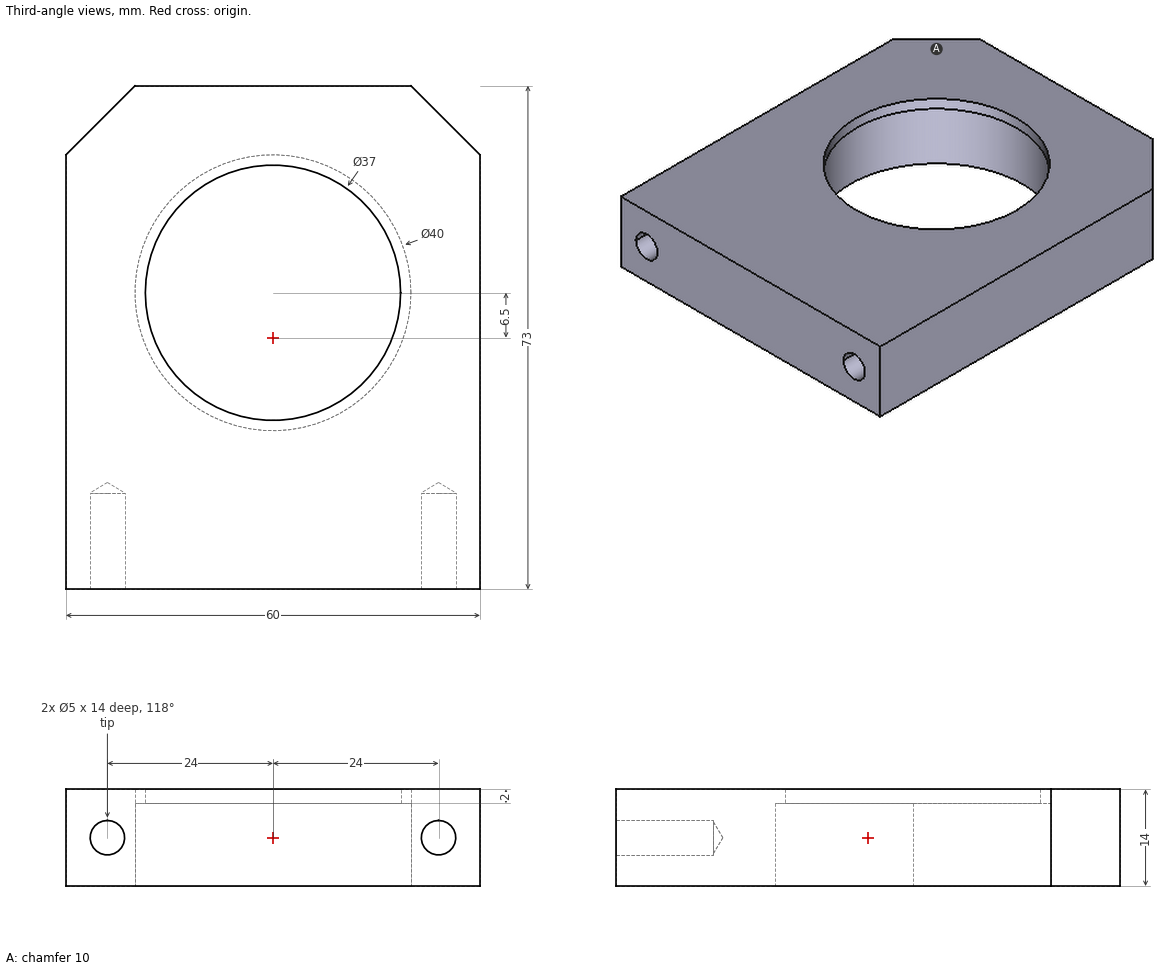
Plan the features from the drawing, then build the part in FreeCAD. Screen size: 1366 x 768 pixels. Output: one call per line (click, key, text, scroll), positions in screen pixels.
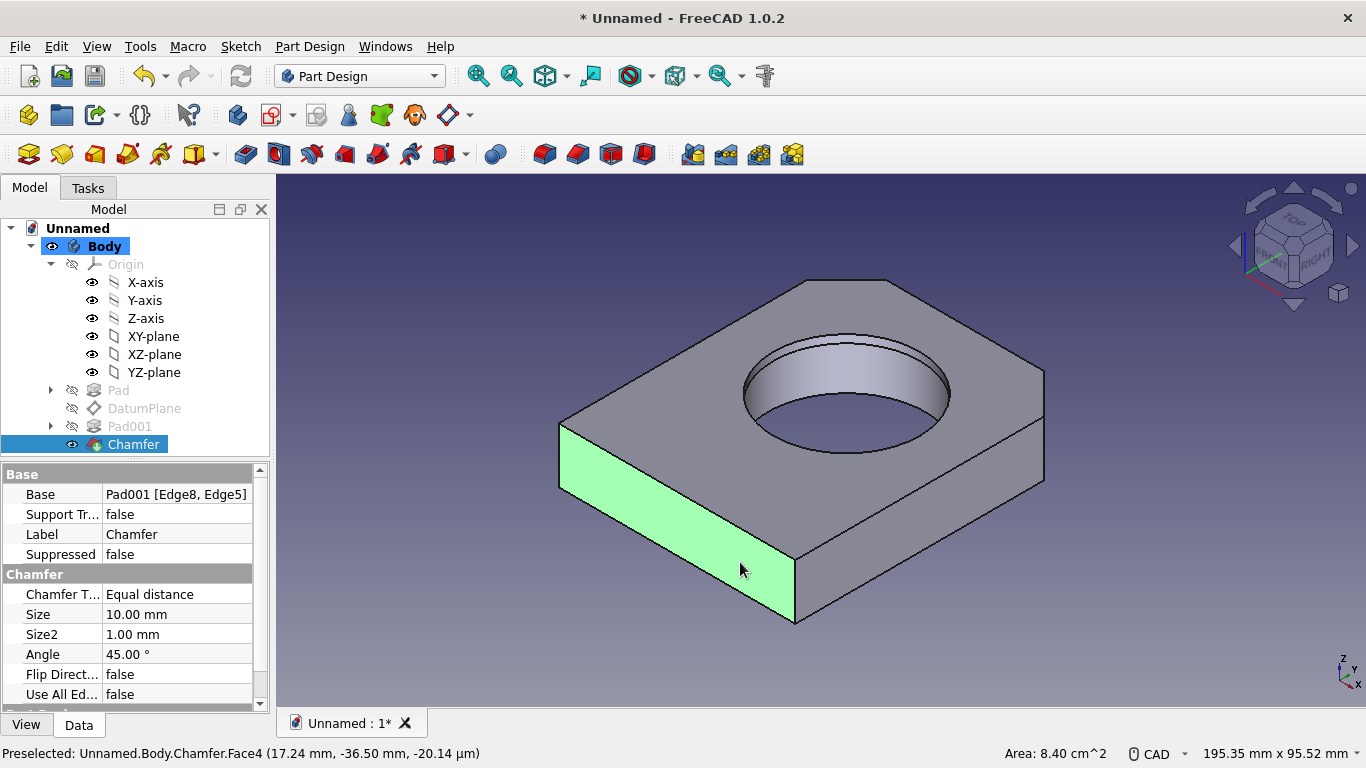
click(270, 116)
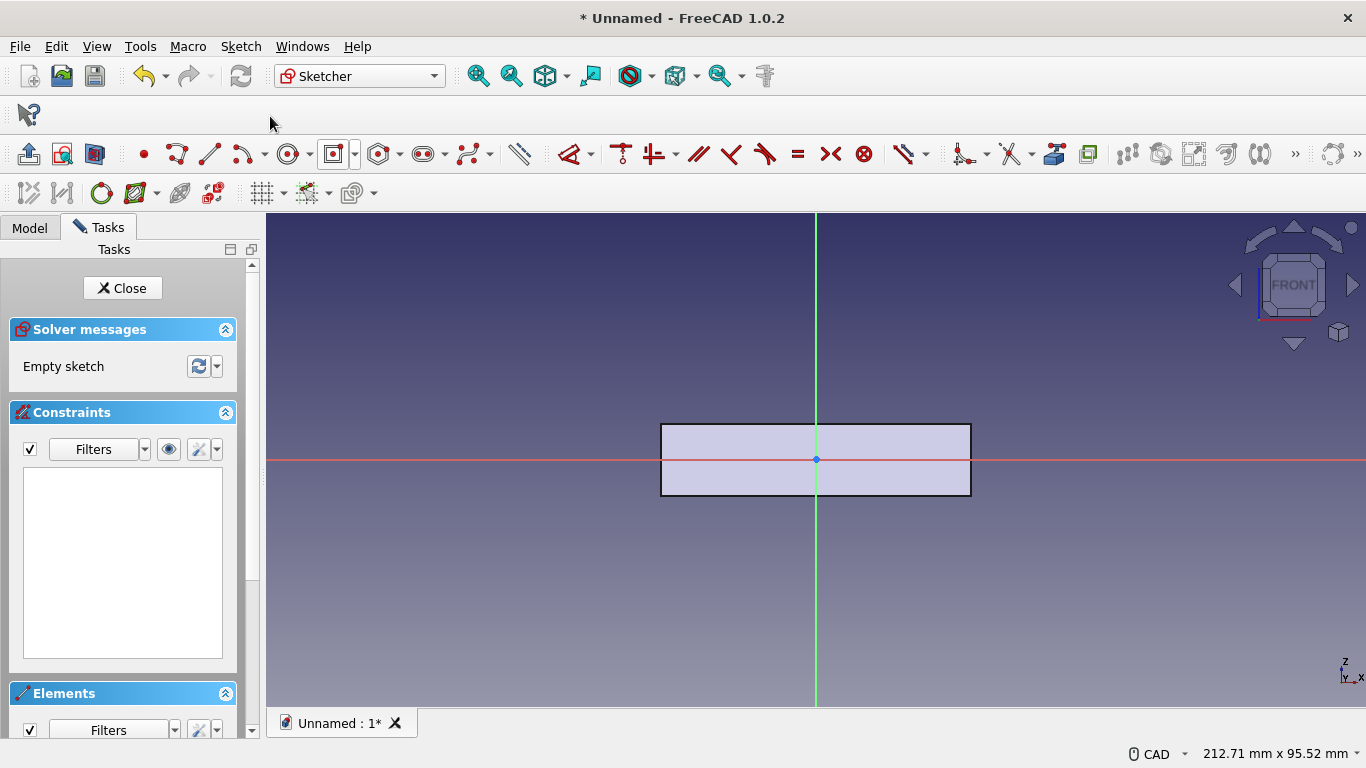
scroll(872, 460, up, 4)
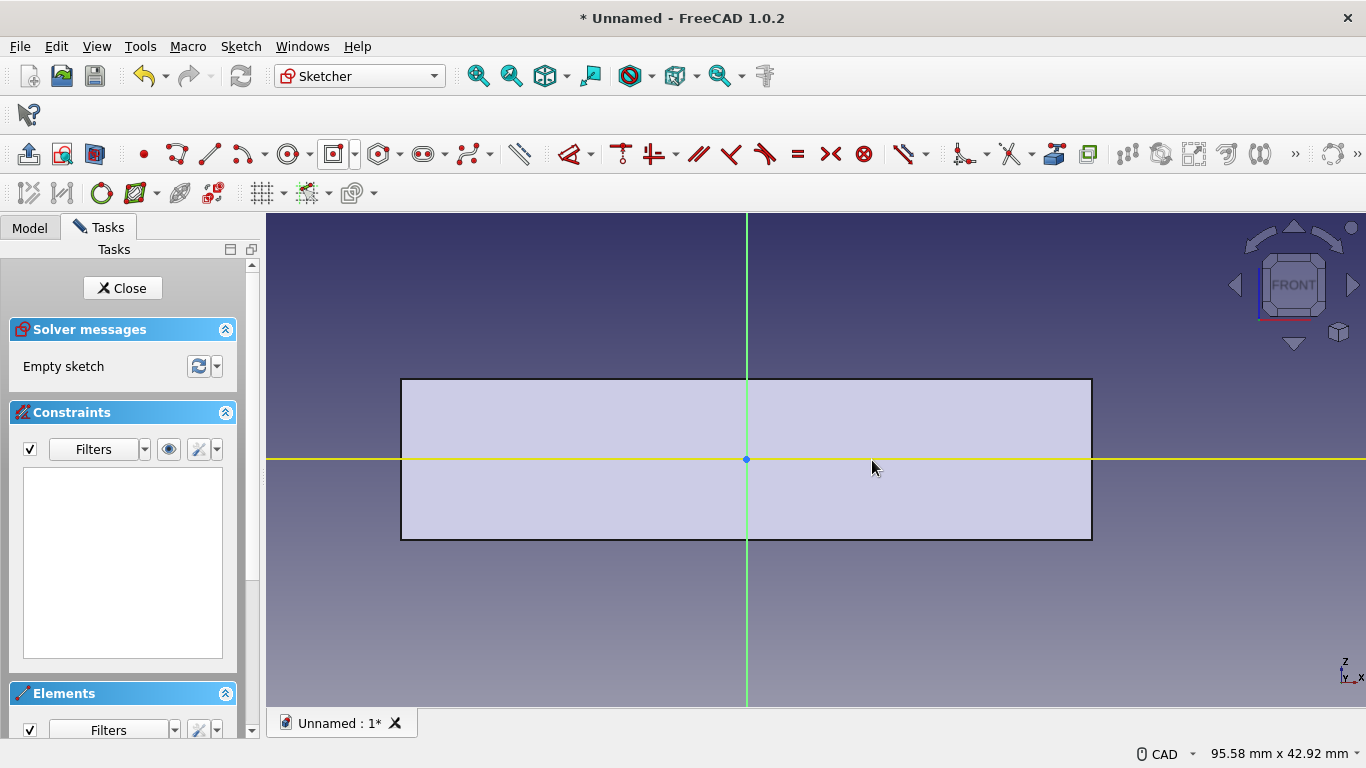
click(288, 154)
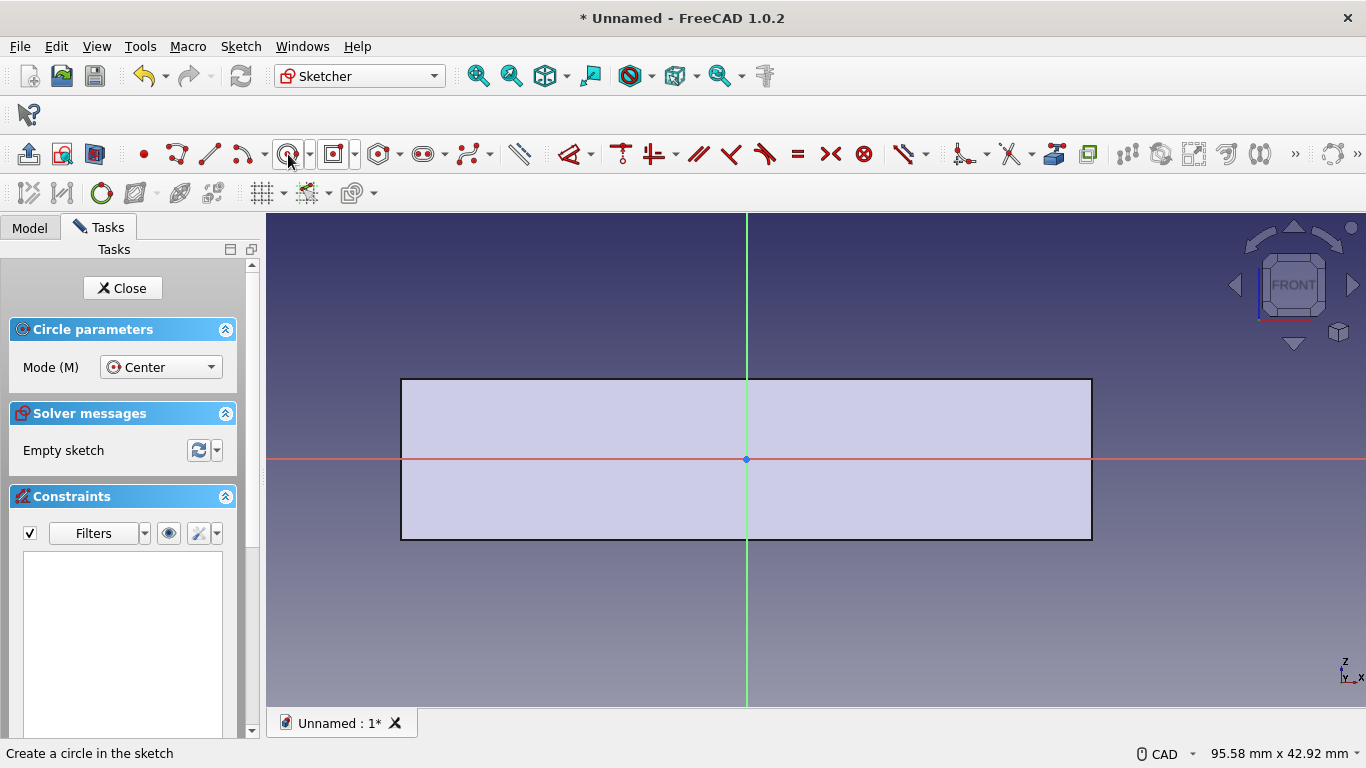
click(470, 459)
move(491, 439)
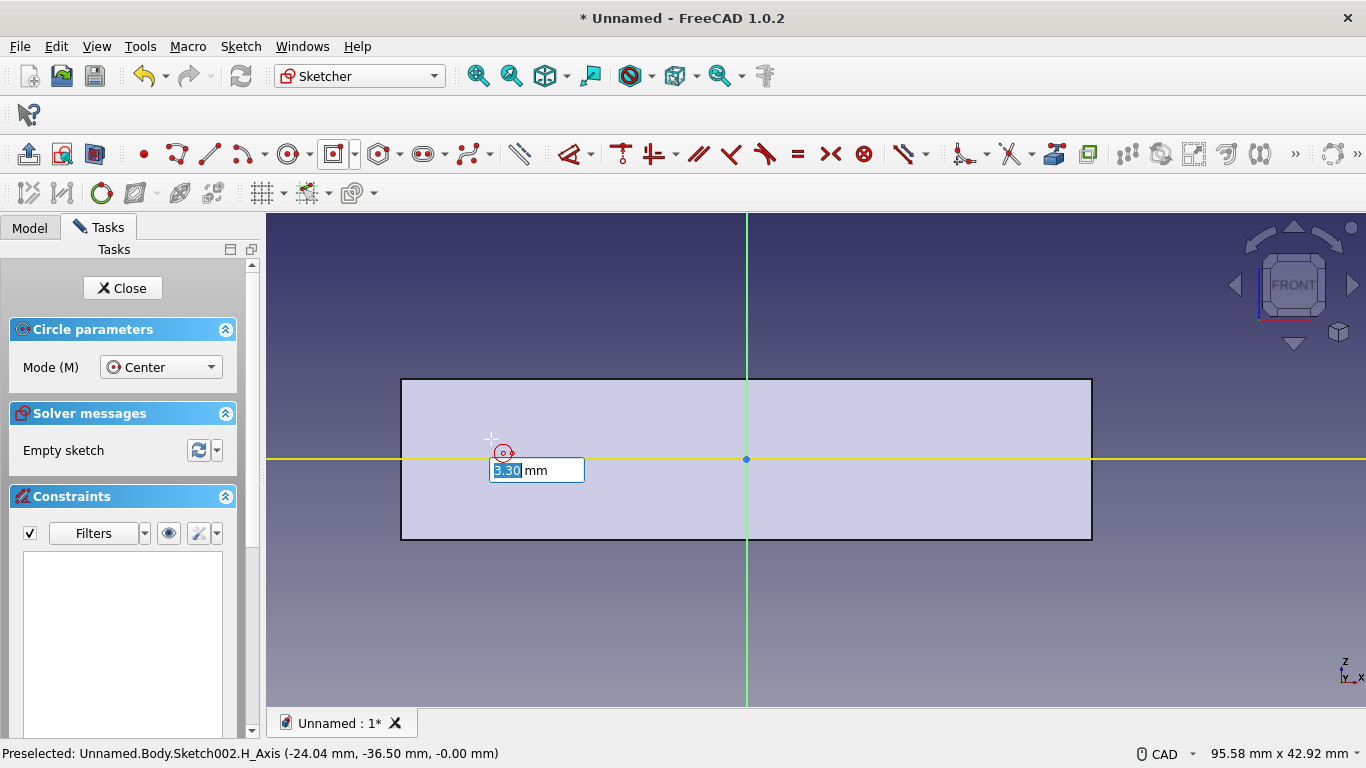
text(5)
key(Return)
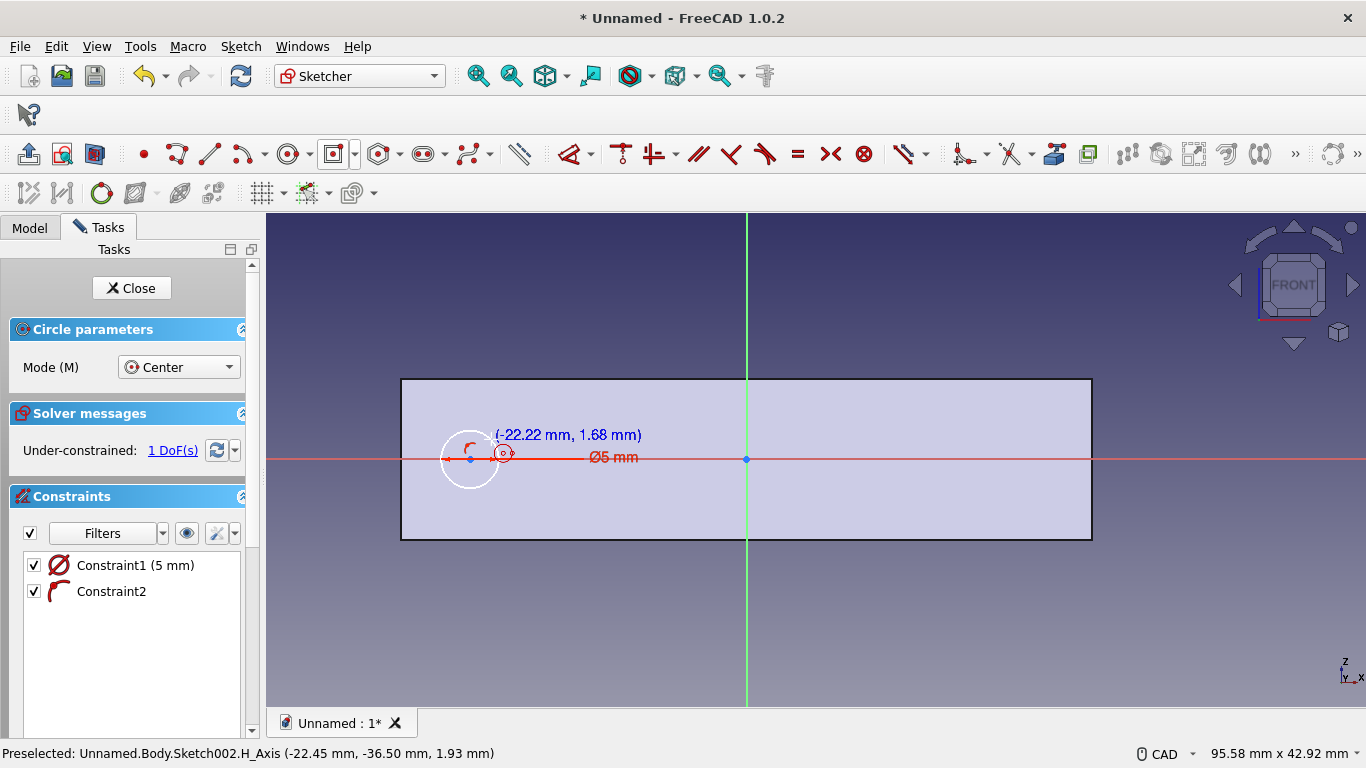
click(1023, 459)
move(1043, 439)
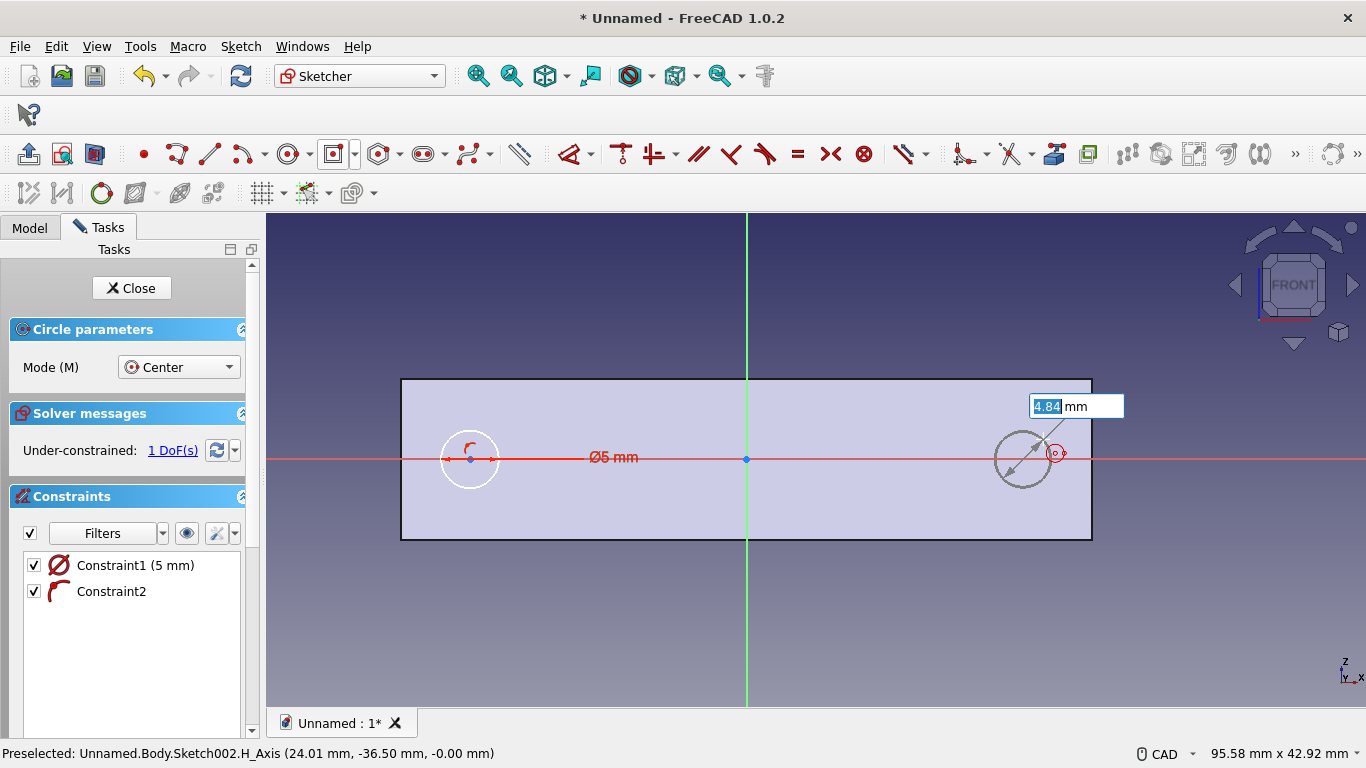
text(5)
key(Return)
key(Escape)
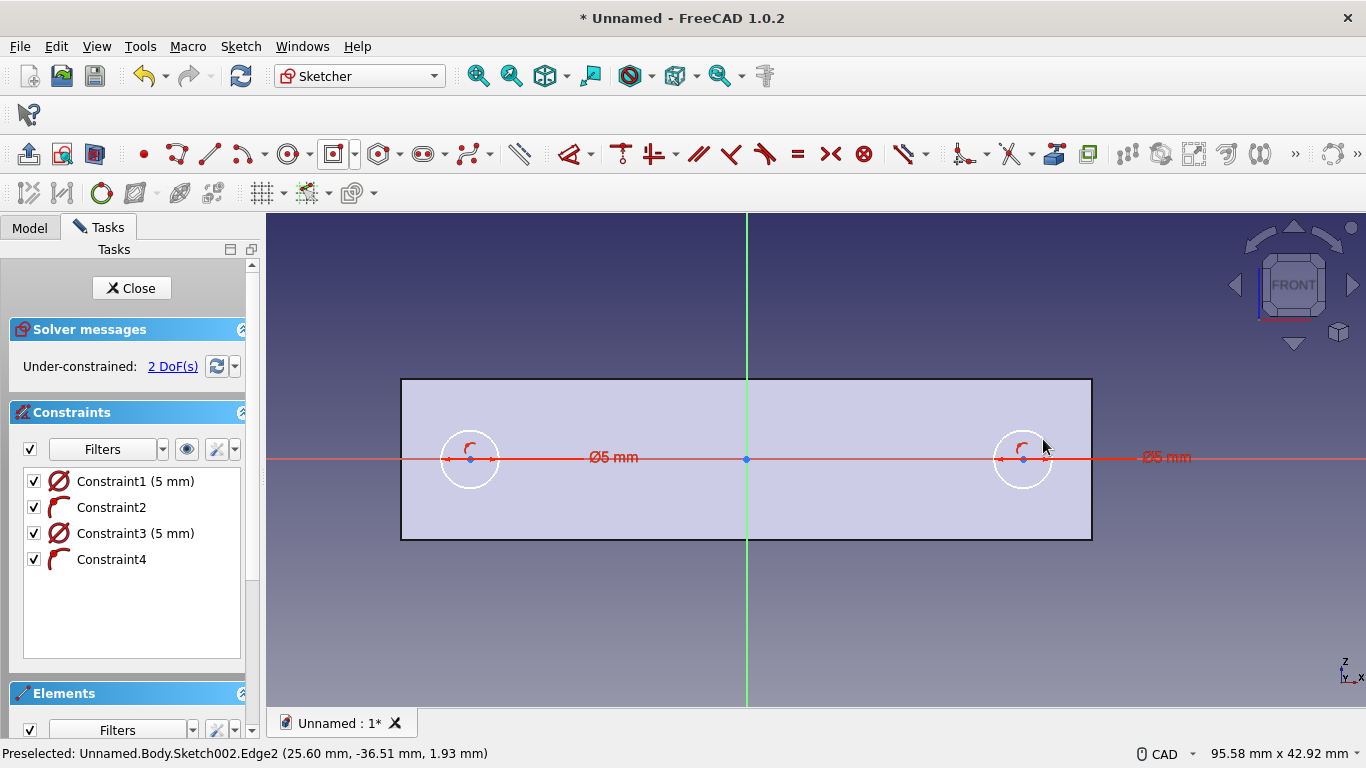
click(568, 154)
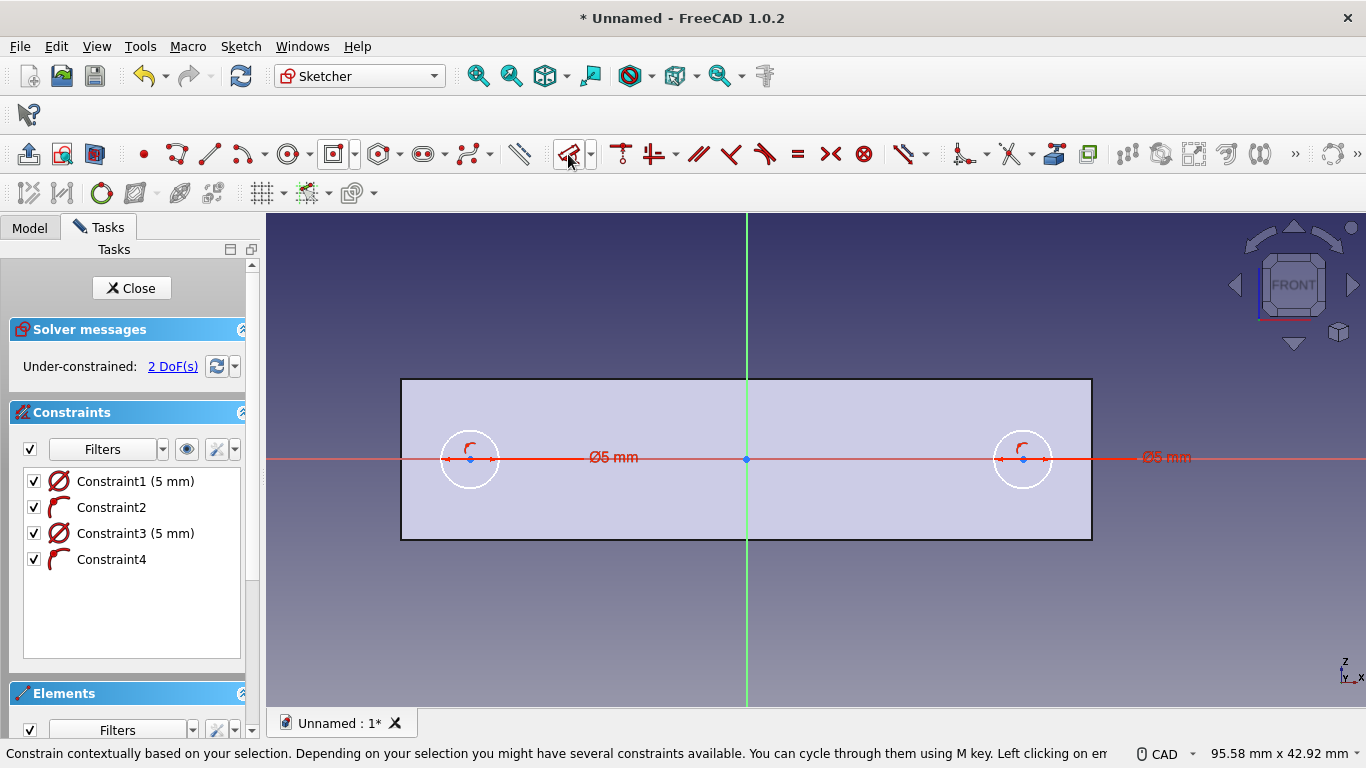
click(470, 459)
click(608, 493)